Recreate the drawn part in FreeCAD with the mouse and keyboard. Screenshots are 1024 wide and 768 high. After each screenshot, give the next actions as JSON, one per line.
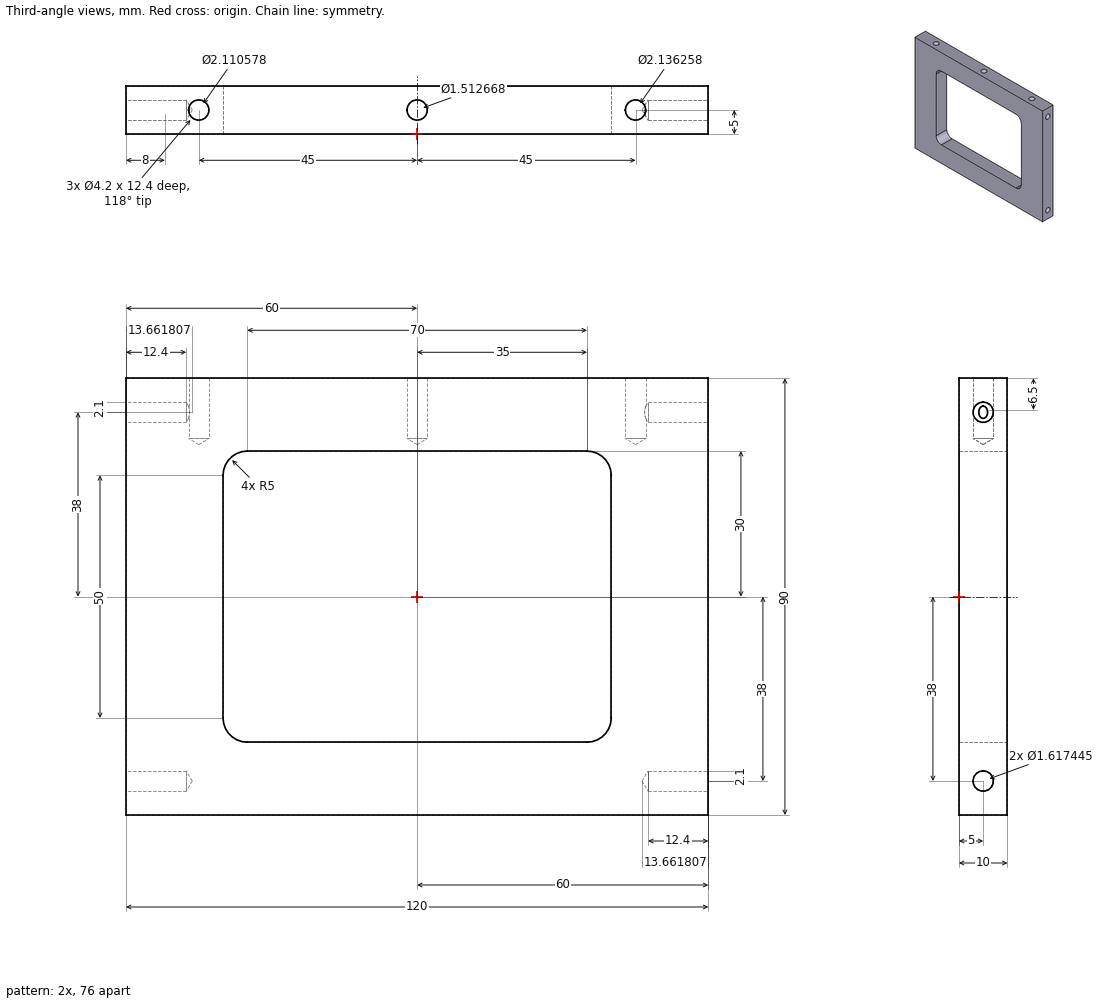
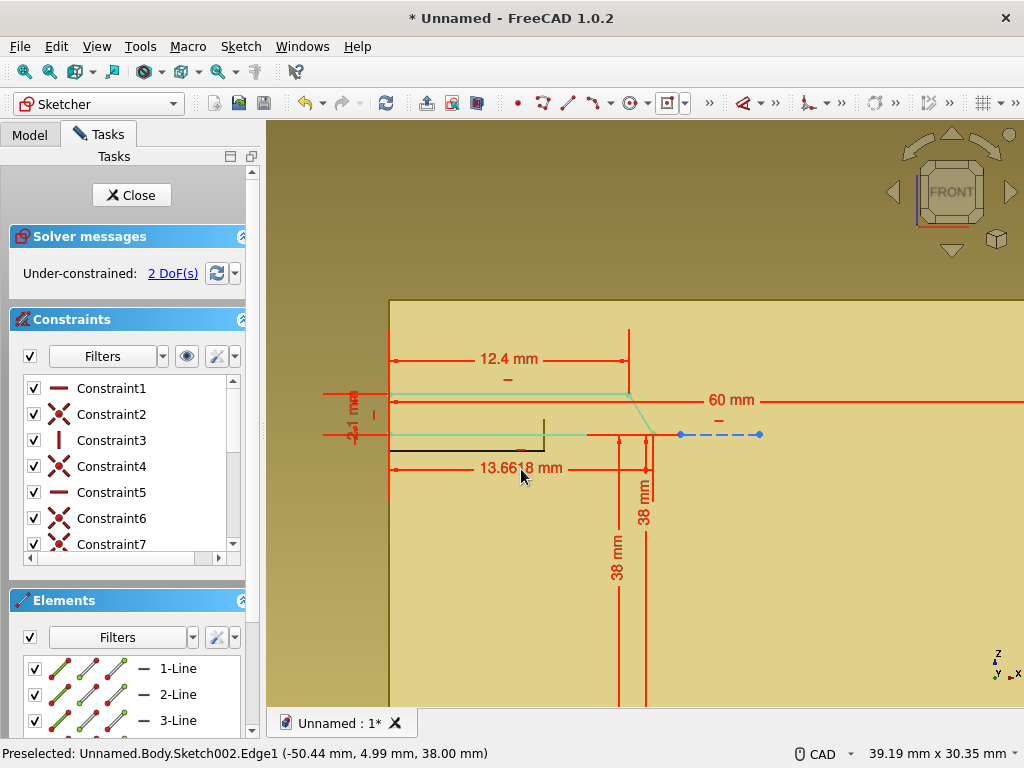
{"action": "left_click", "coordinate": [132, 195]}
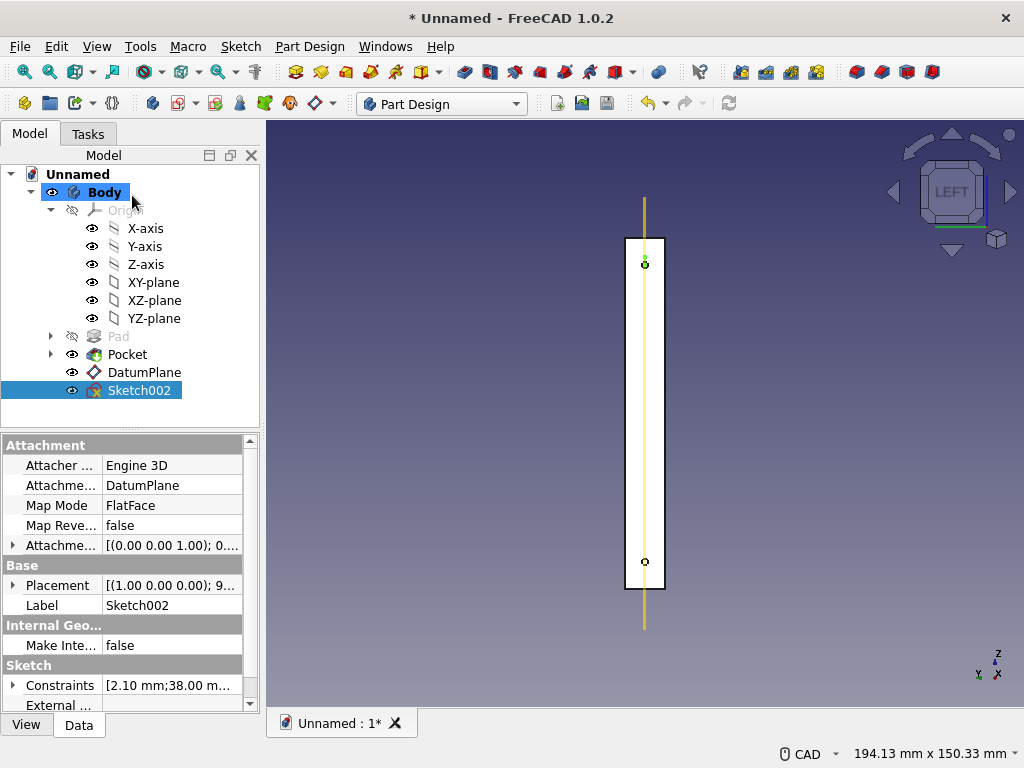
{"action": "left_click", "coordinate": [515, 72]}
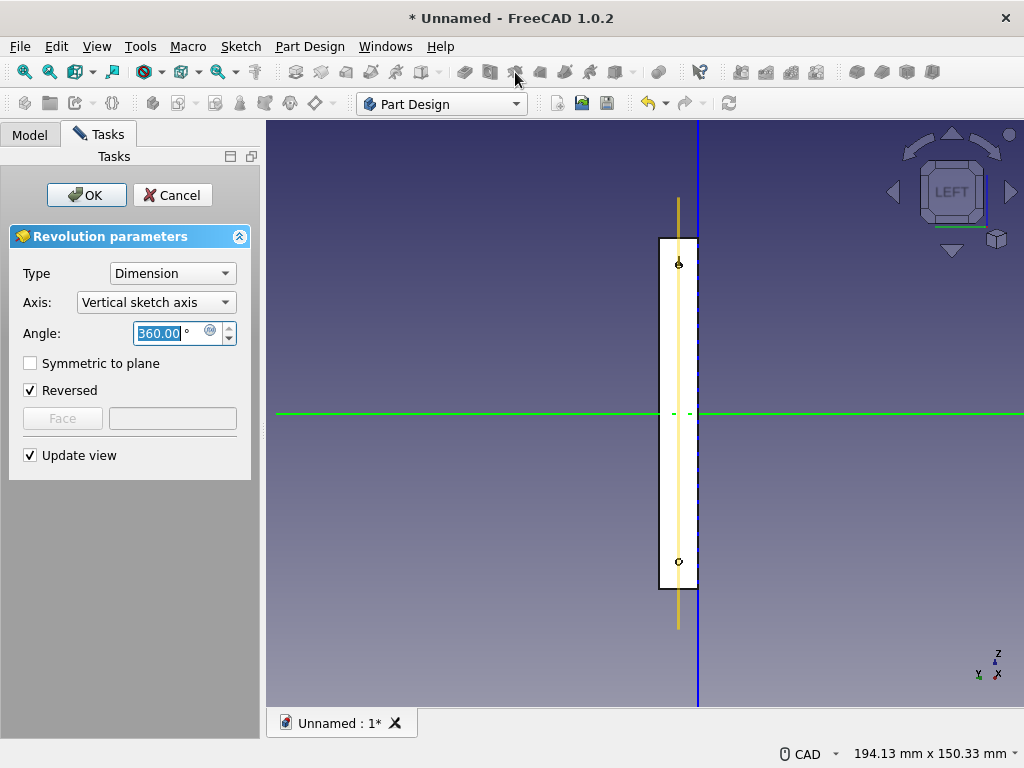
{"action": "left_click", "coordinate": [157, 302]}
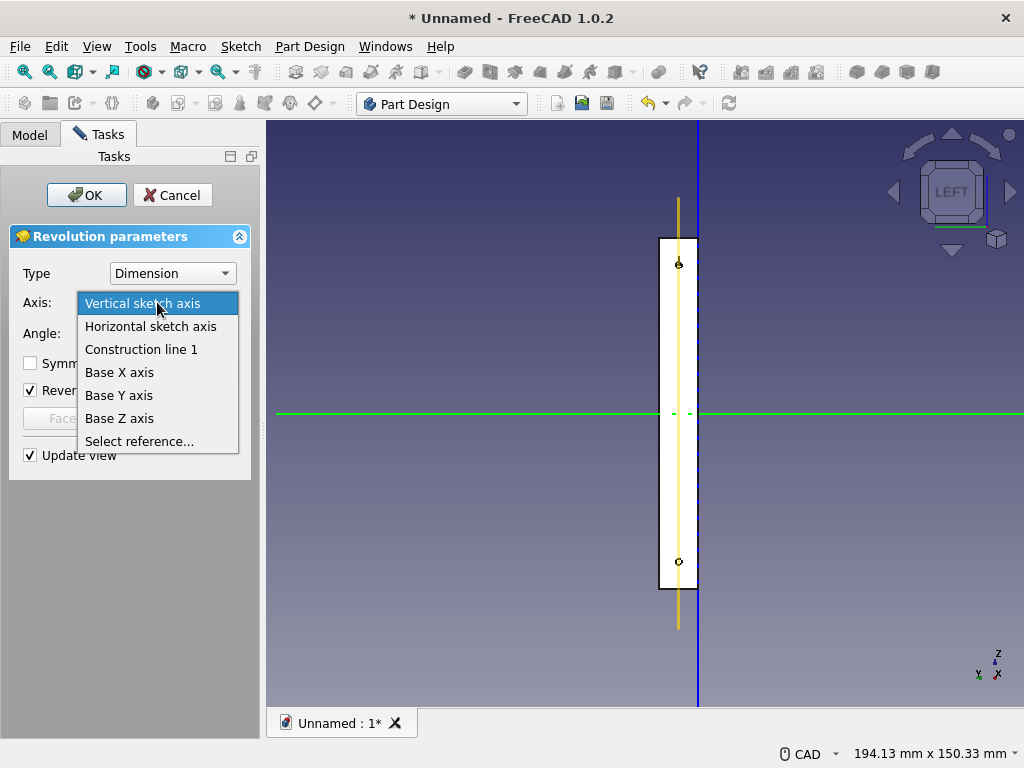
{"action": "left_click", "coordinate": [156, 350]}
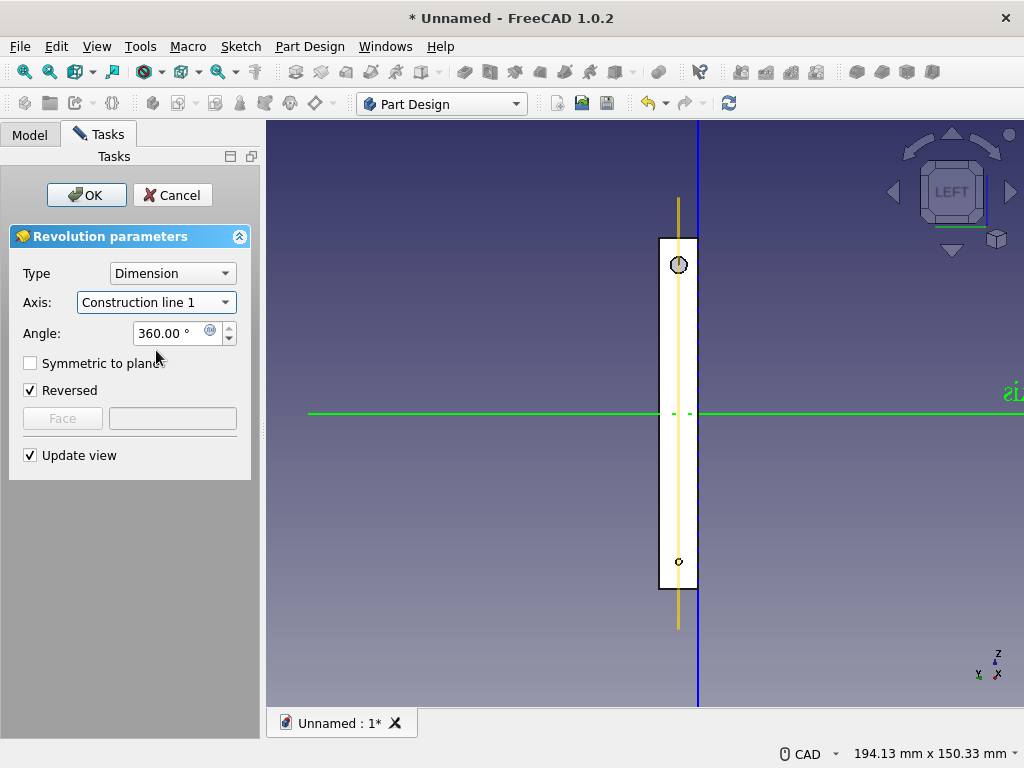
{"action": "left_click", "coordinate": [87, 195]}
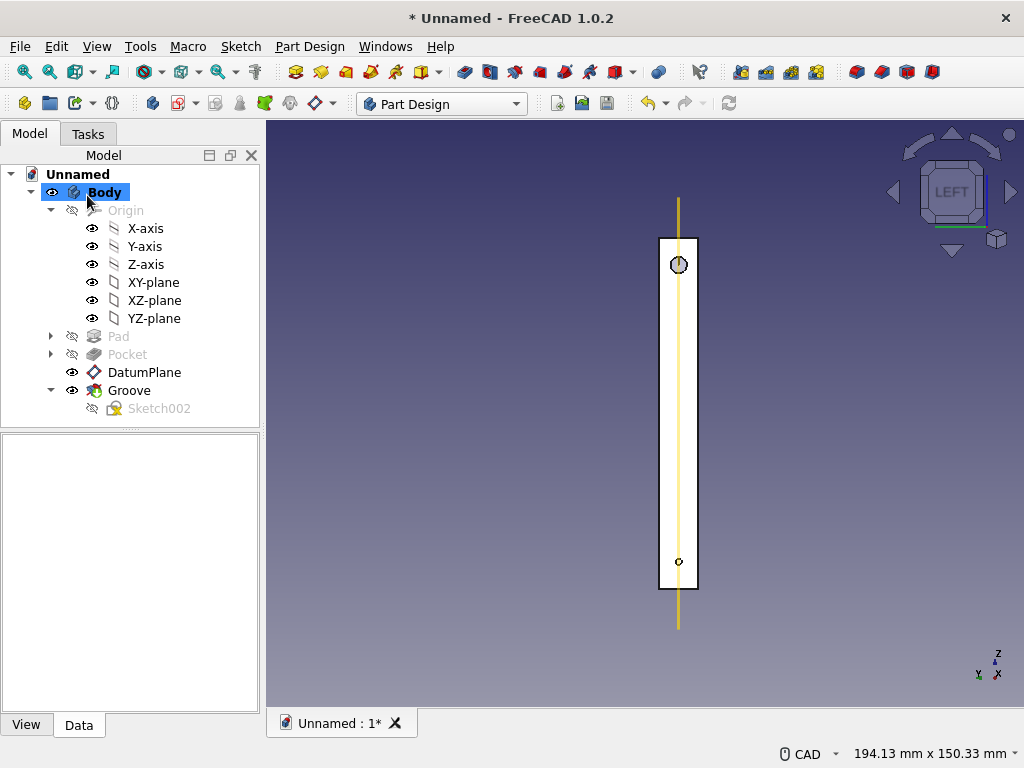
{"action": "left_click", "coordinate": [117, 372]}
{"action": "key", "text": "space"}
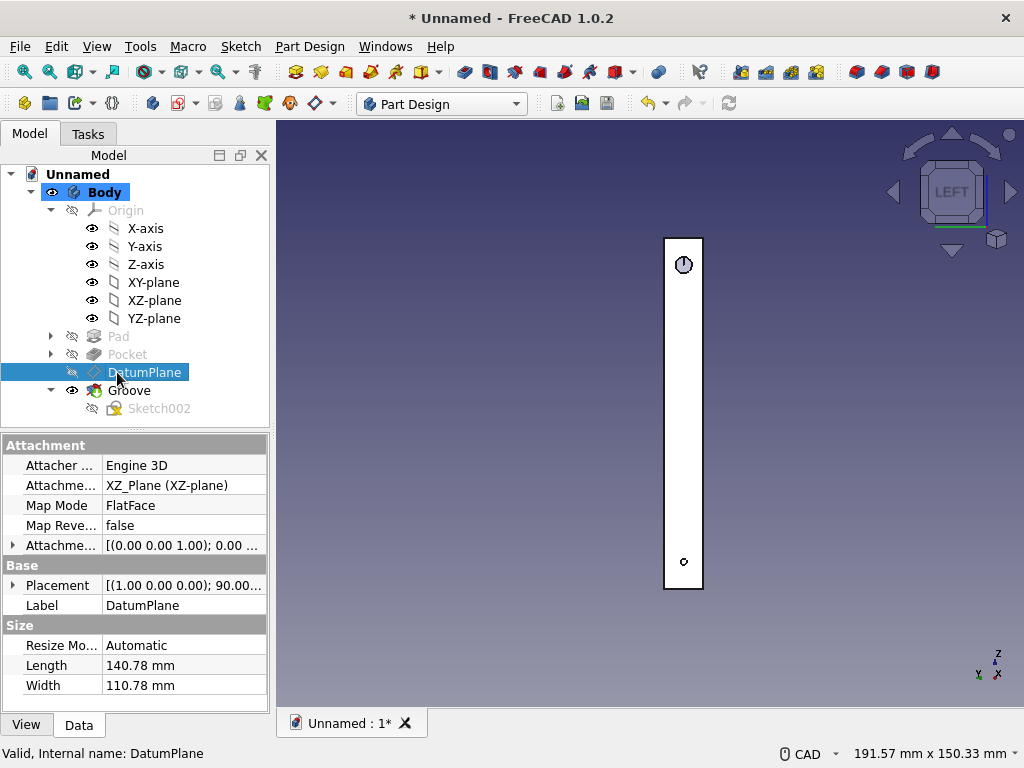
{"action": "left_click", "coordinate": [117, 390]}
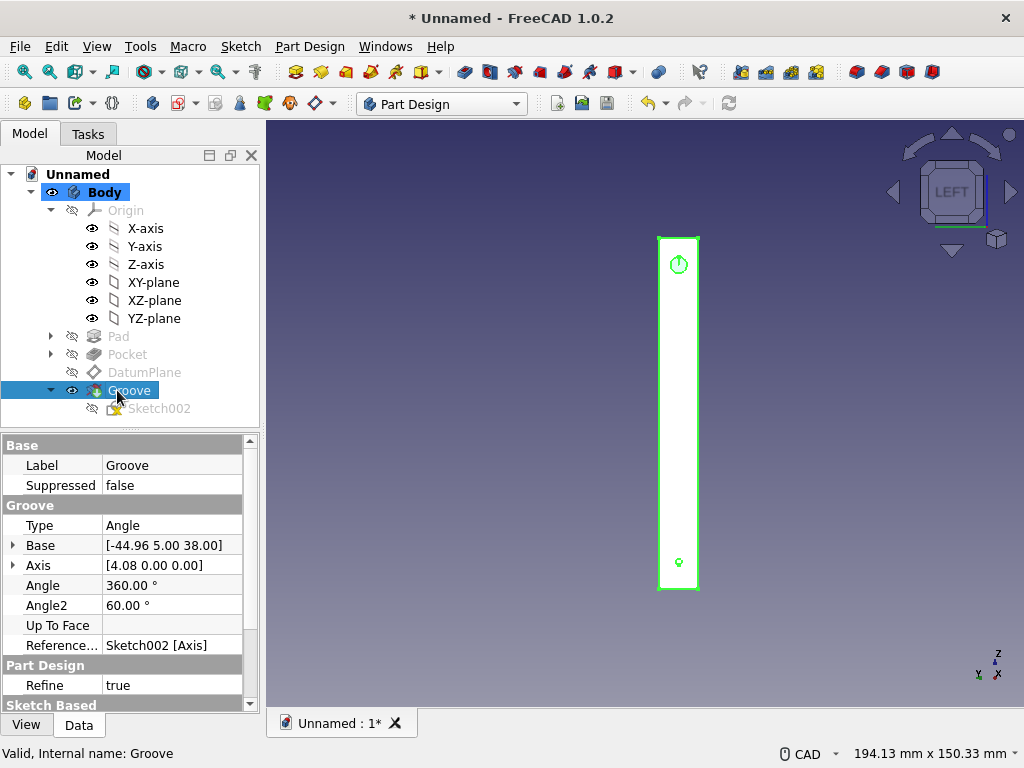
{"action": "left_click", "coordinate": [766, 72]}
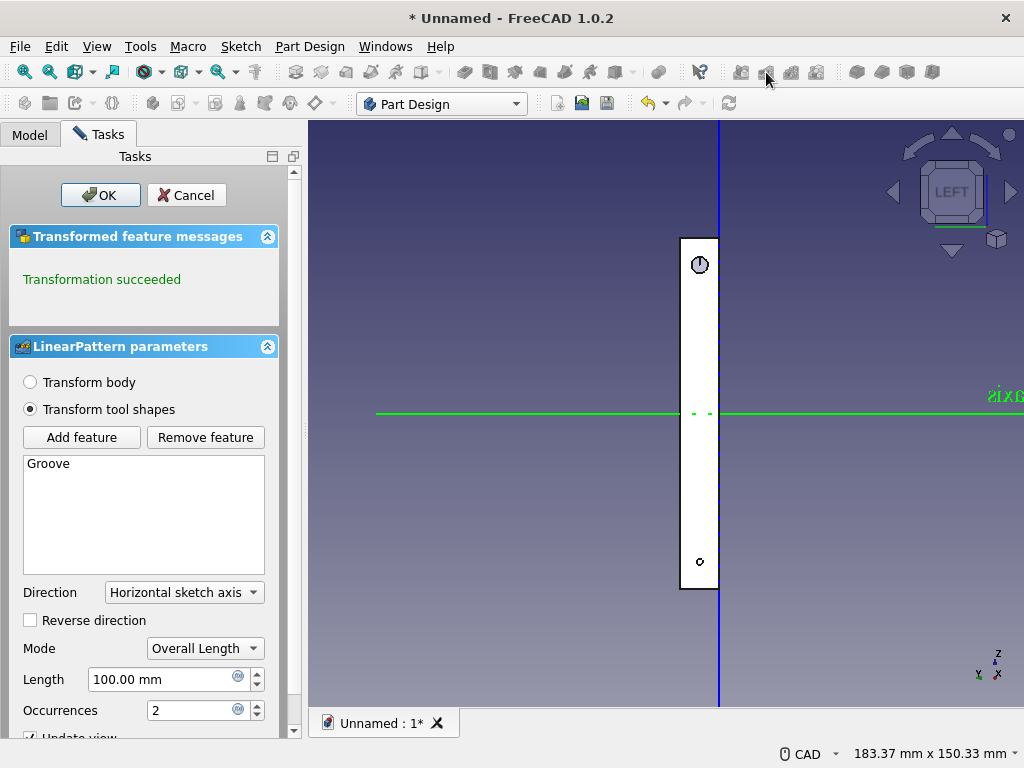
{"action": "left_click", "coordinate": [185, 592]}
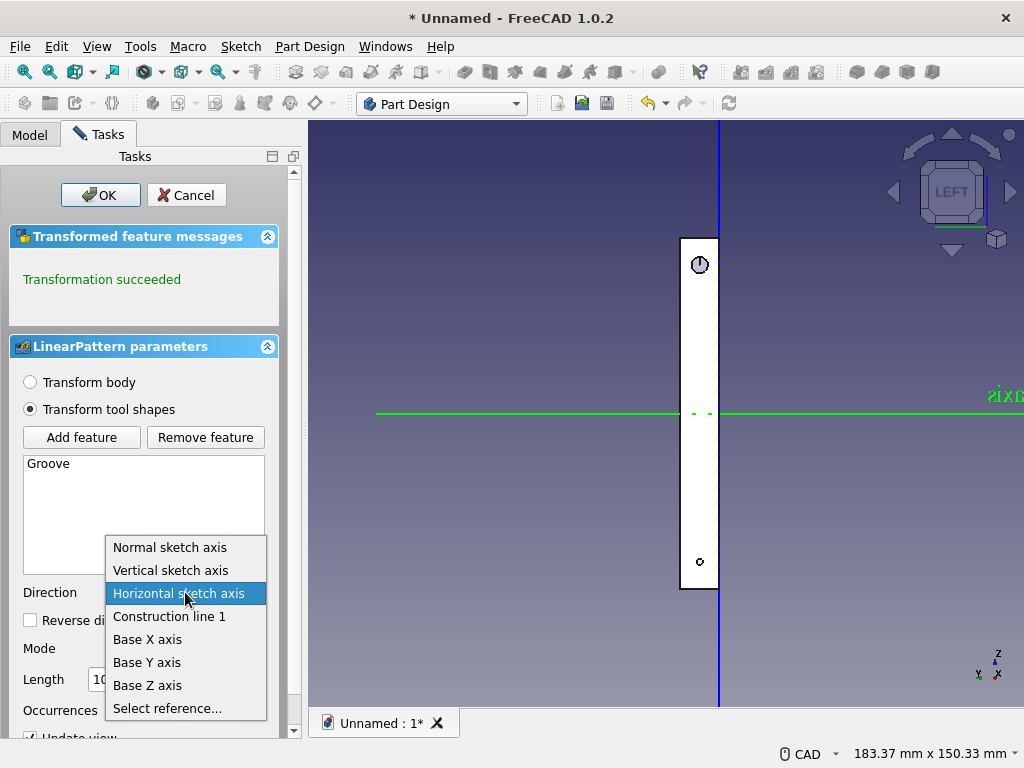
{"action": "left_click", "coordinate": [184, 686]}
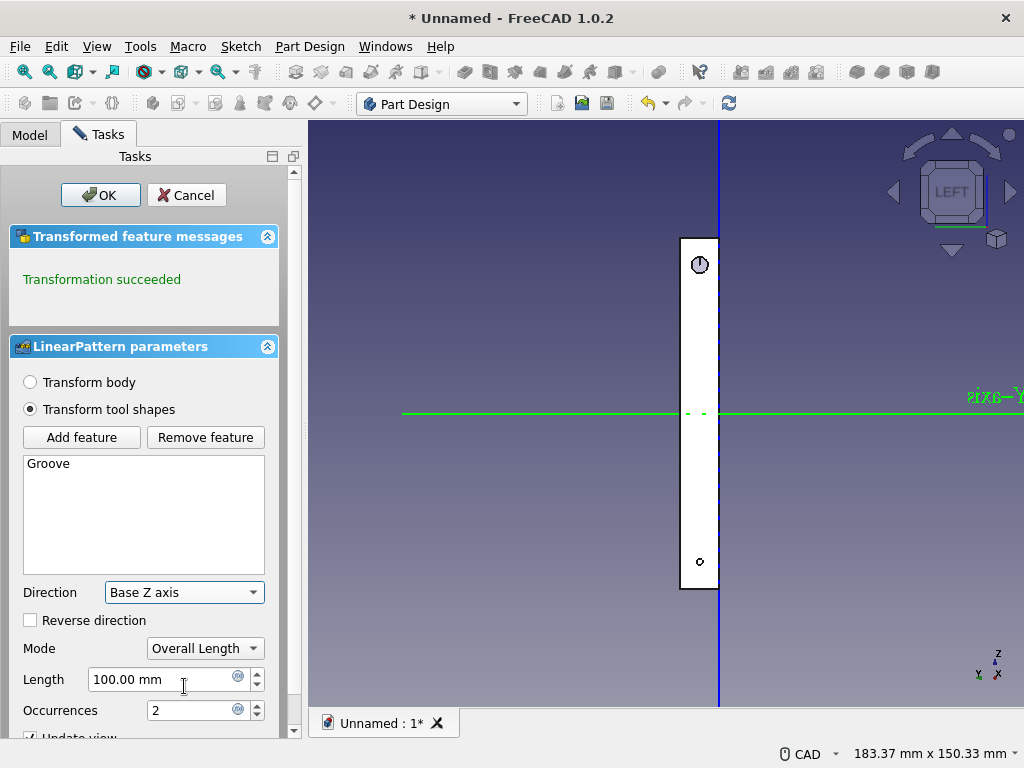
{"action": "left_click", "coordinate": [206, 648]}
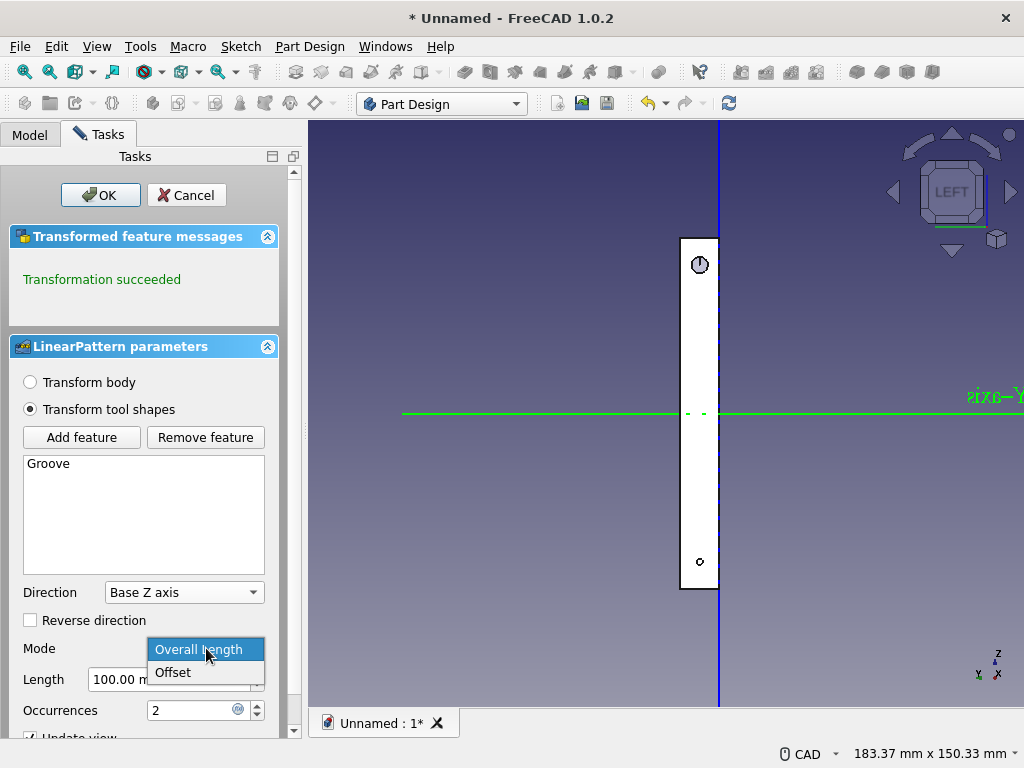
{"action": "left_click", "coordinate": [204, 672]}